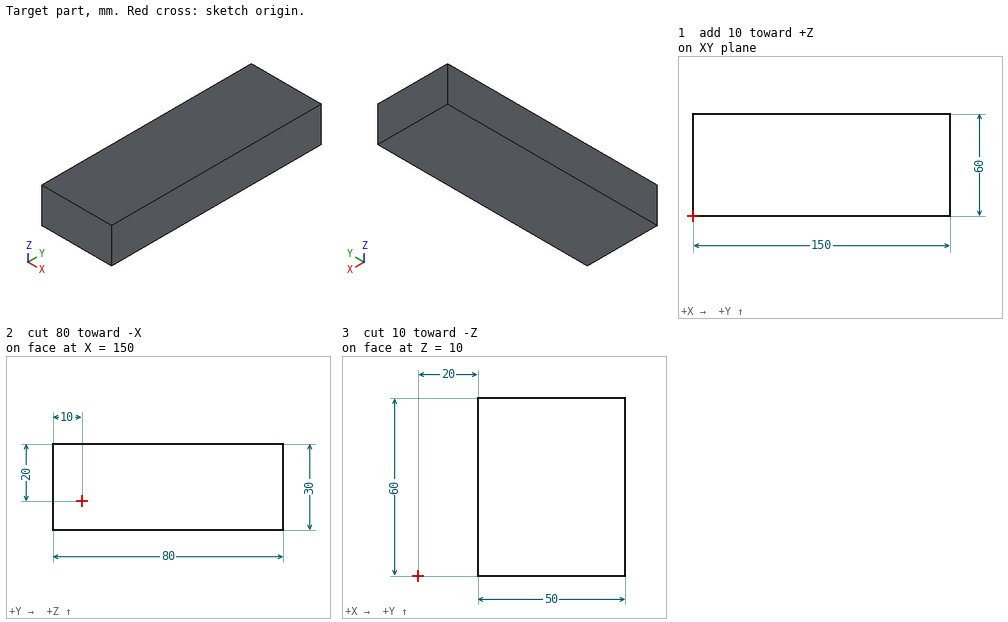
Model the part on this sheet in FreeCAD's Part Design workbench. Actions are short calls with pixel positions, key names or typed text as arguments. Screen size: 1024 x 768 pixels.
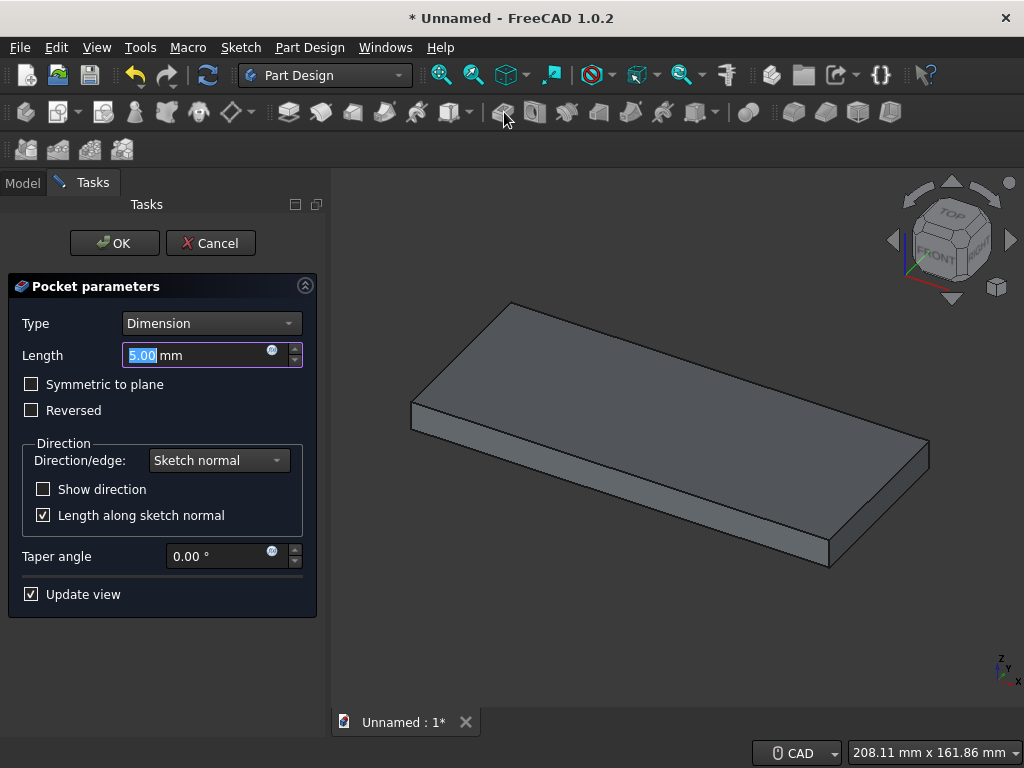
text(80)
key(Tab)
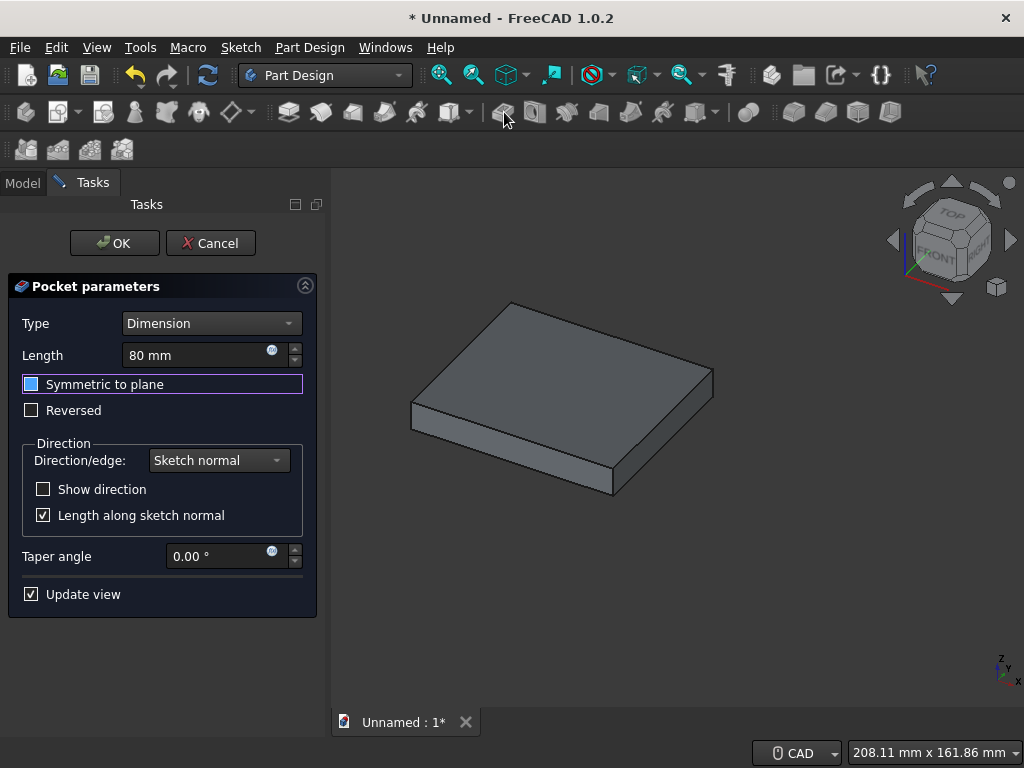
click(115, 243)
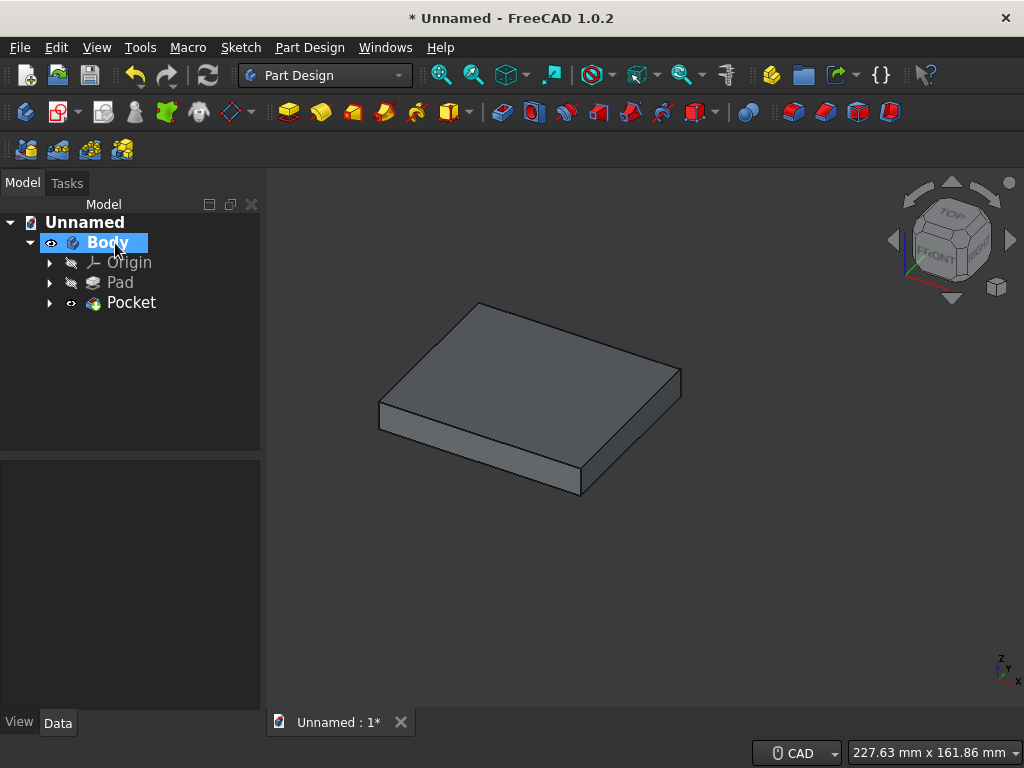
click(442, 76)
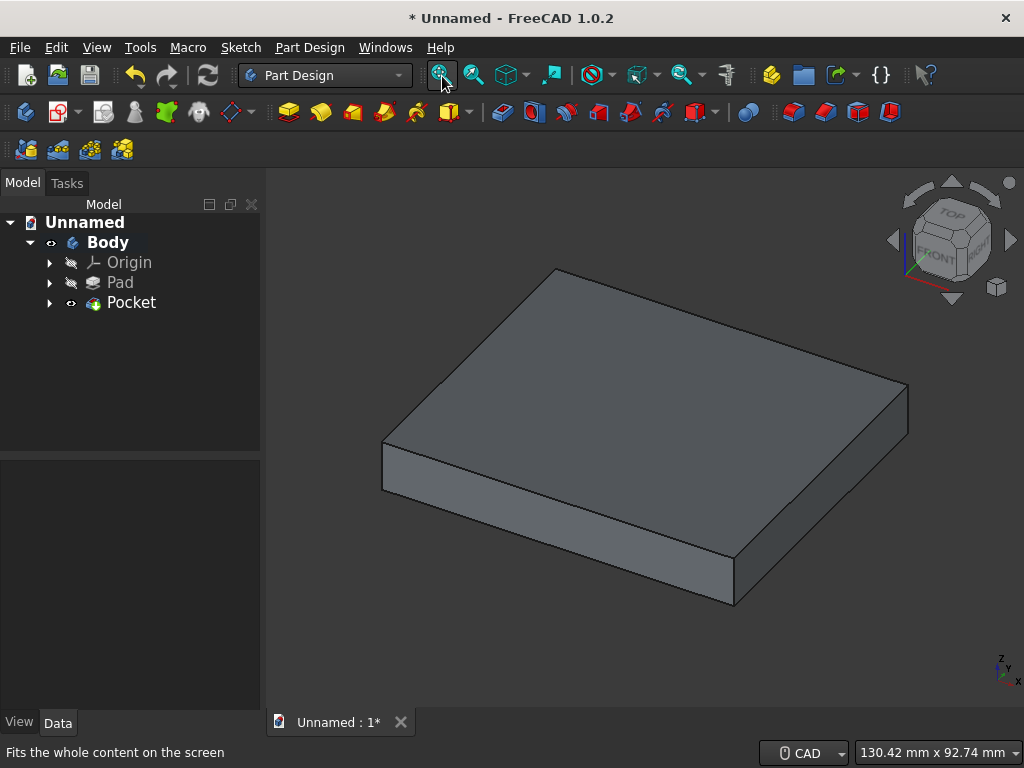
click(645, 413)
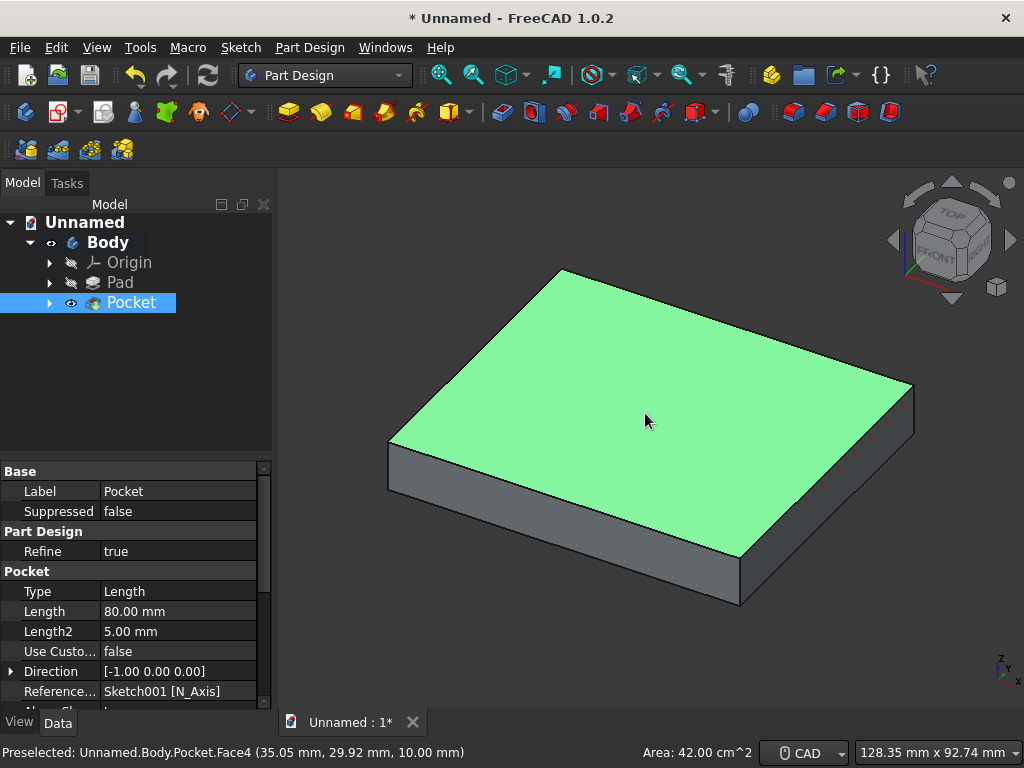
click(58, 112)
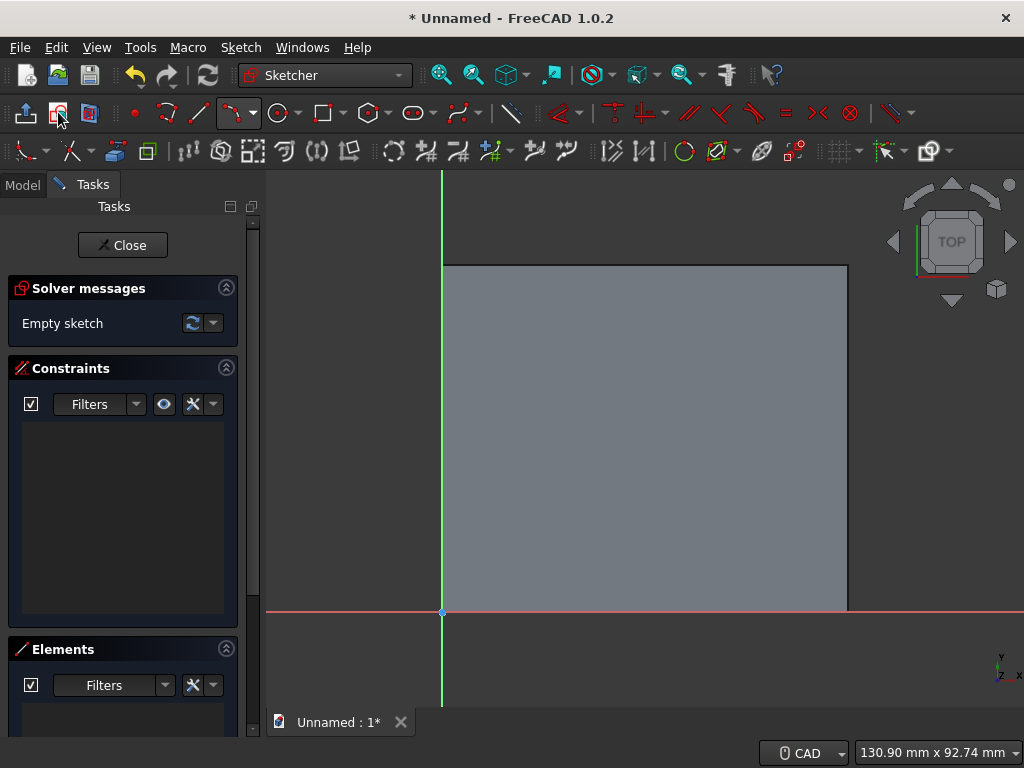
scroll(294, 439, down, 1)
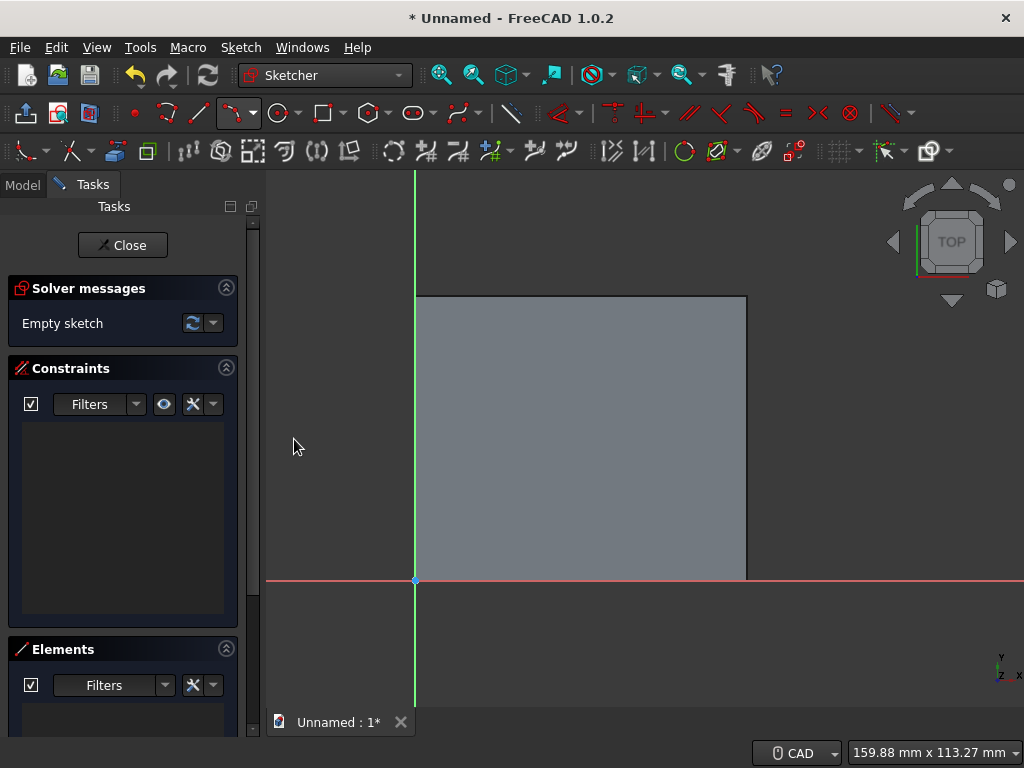
click(324, 114)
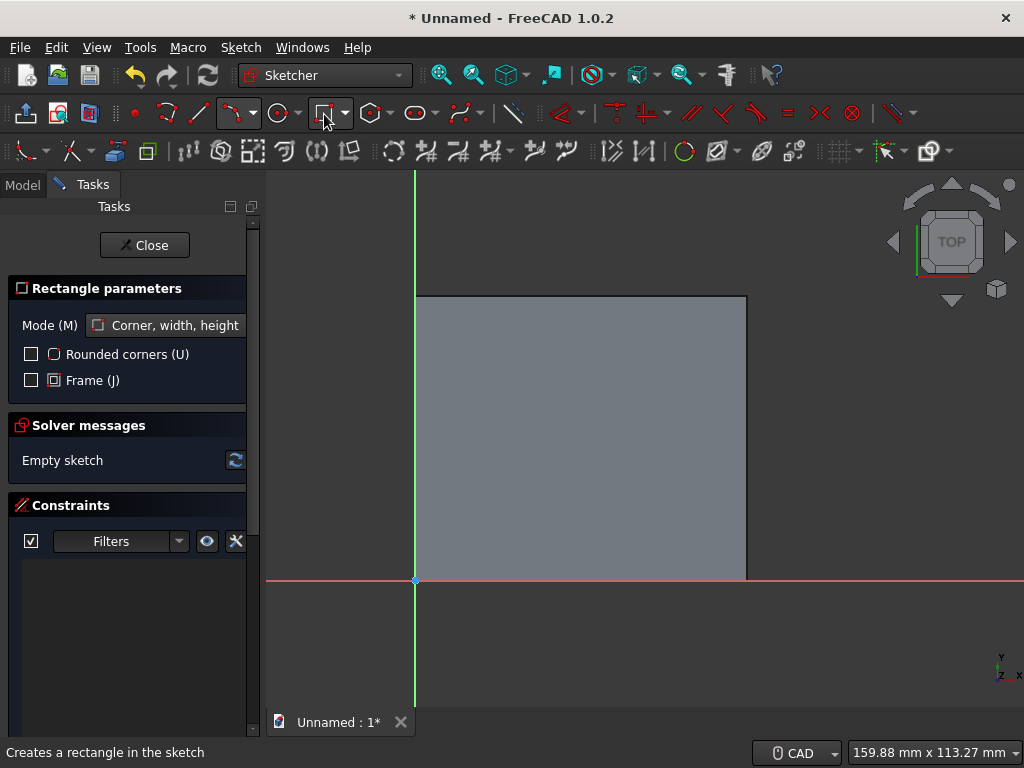
click(510, 296)
click(747, 581)
key(Escape)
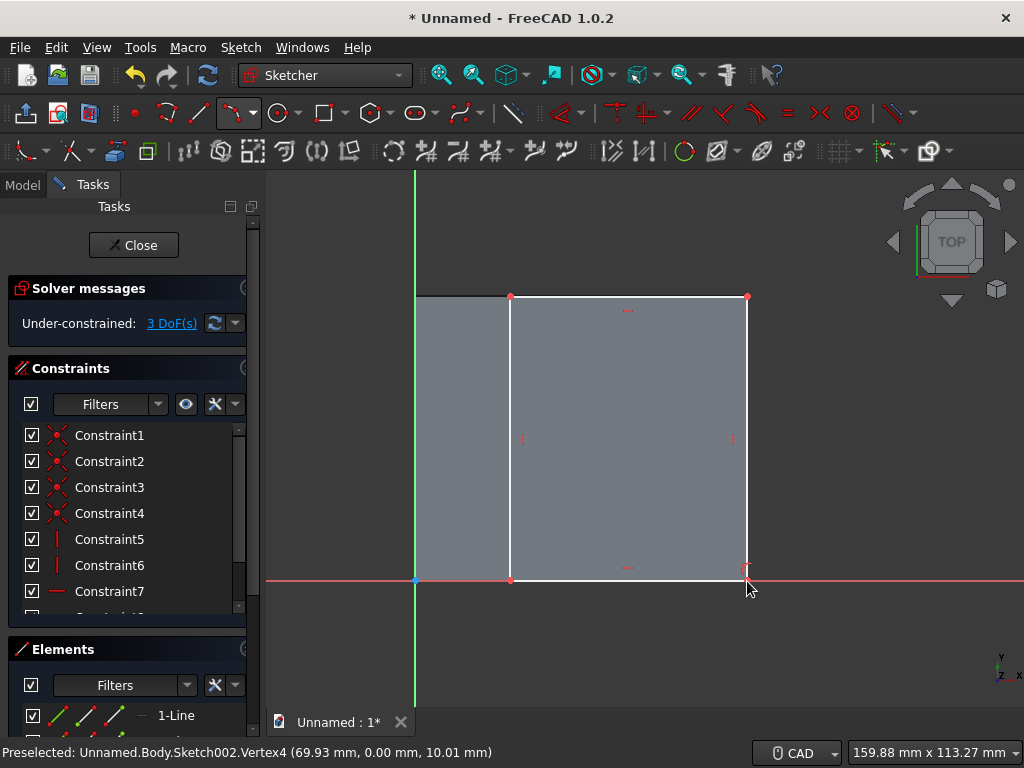
click(560, 114)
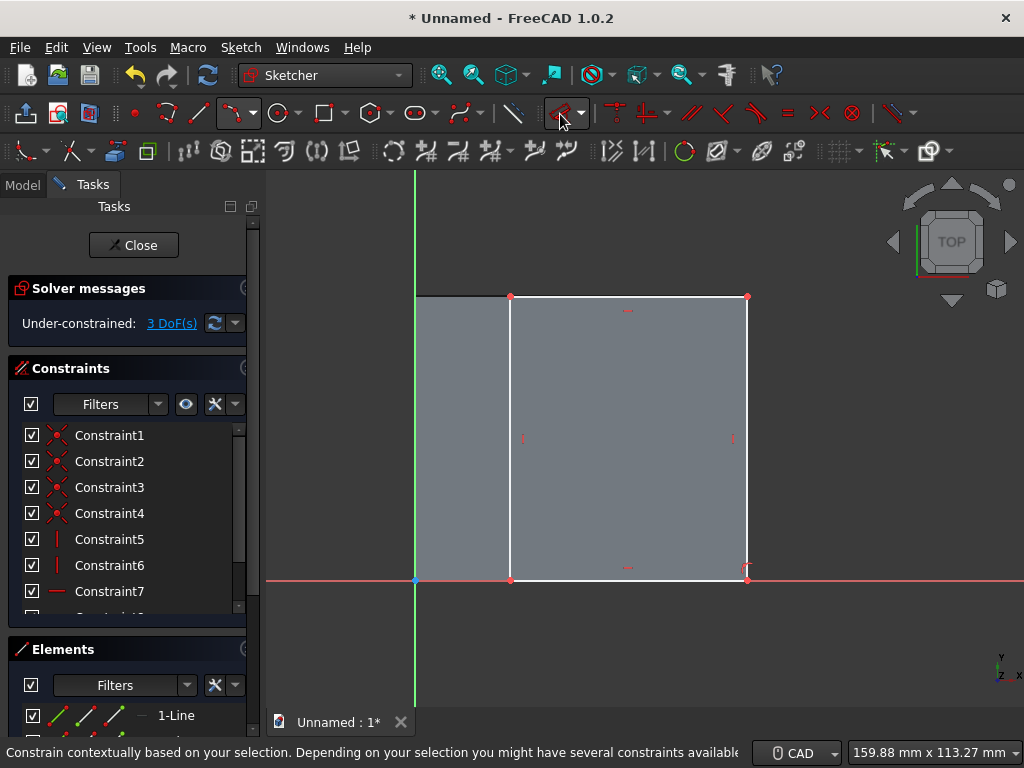
click(510, 382)
click(476, 439)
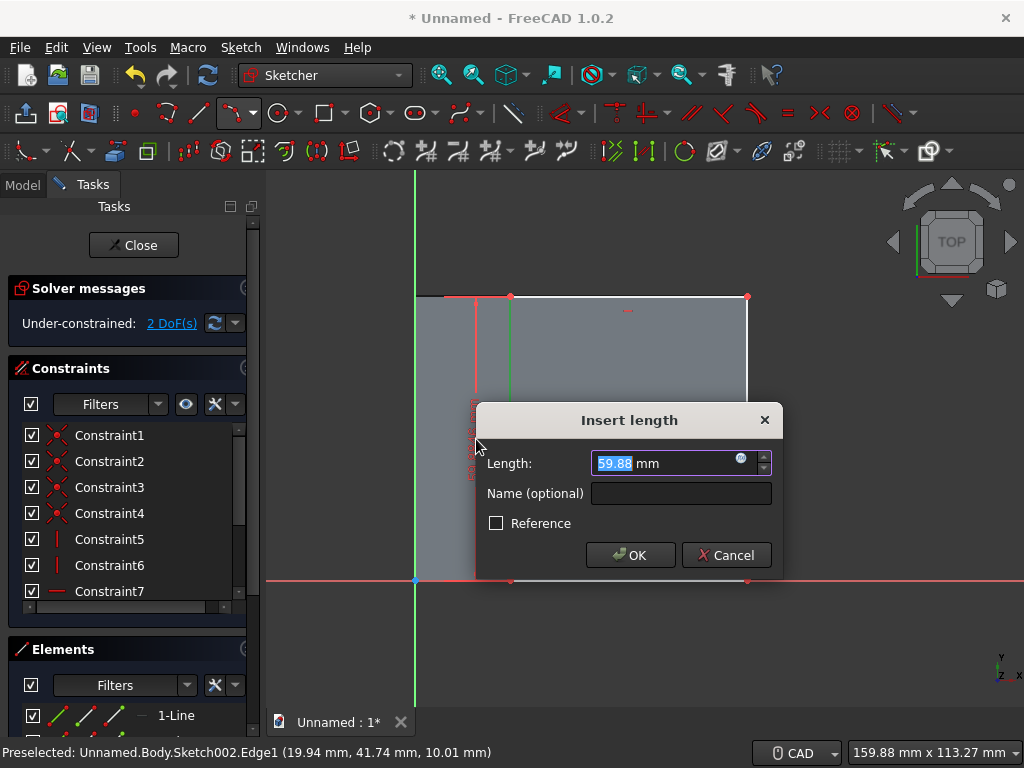
text(60)
key(Return)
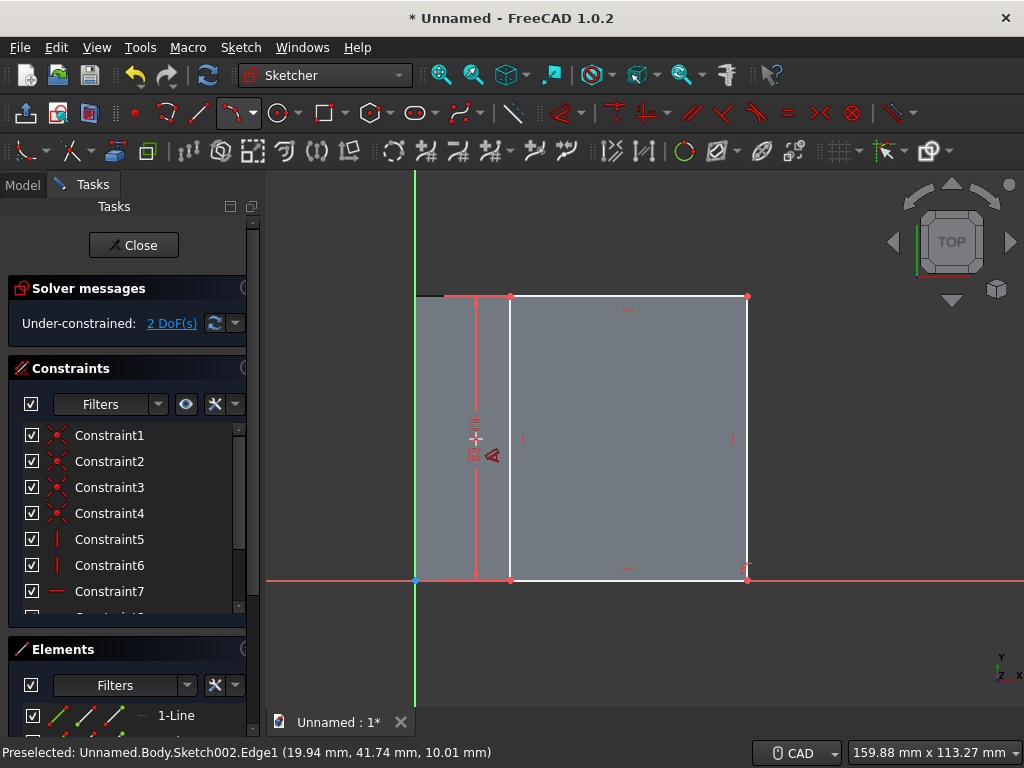
click(581, 581)
click(628, 615)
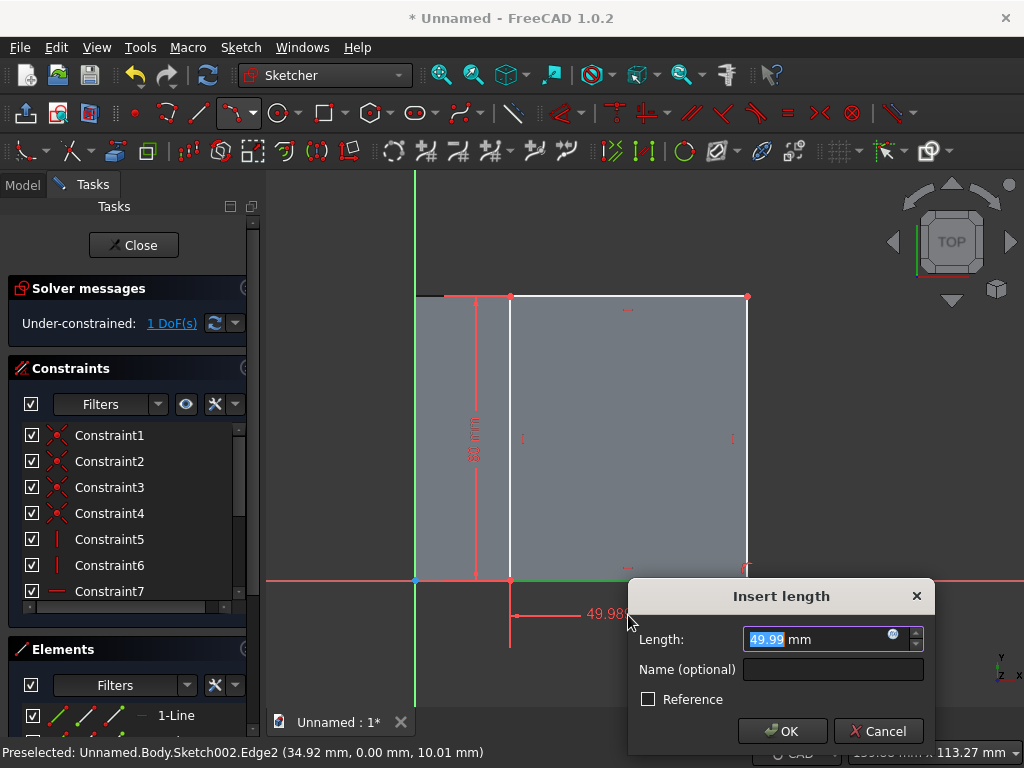
text(50)
key(Return)